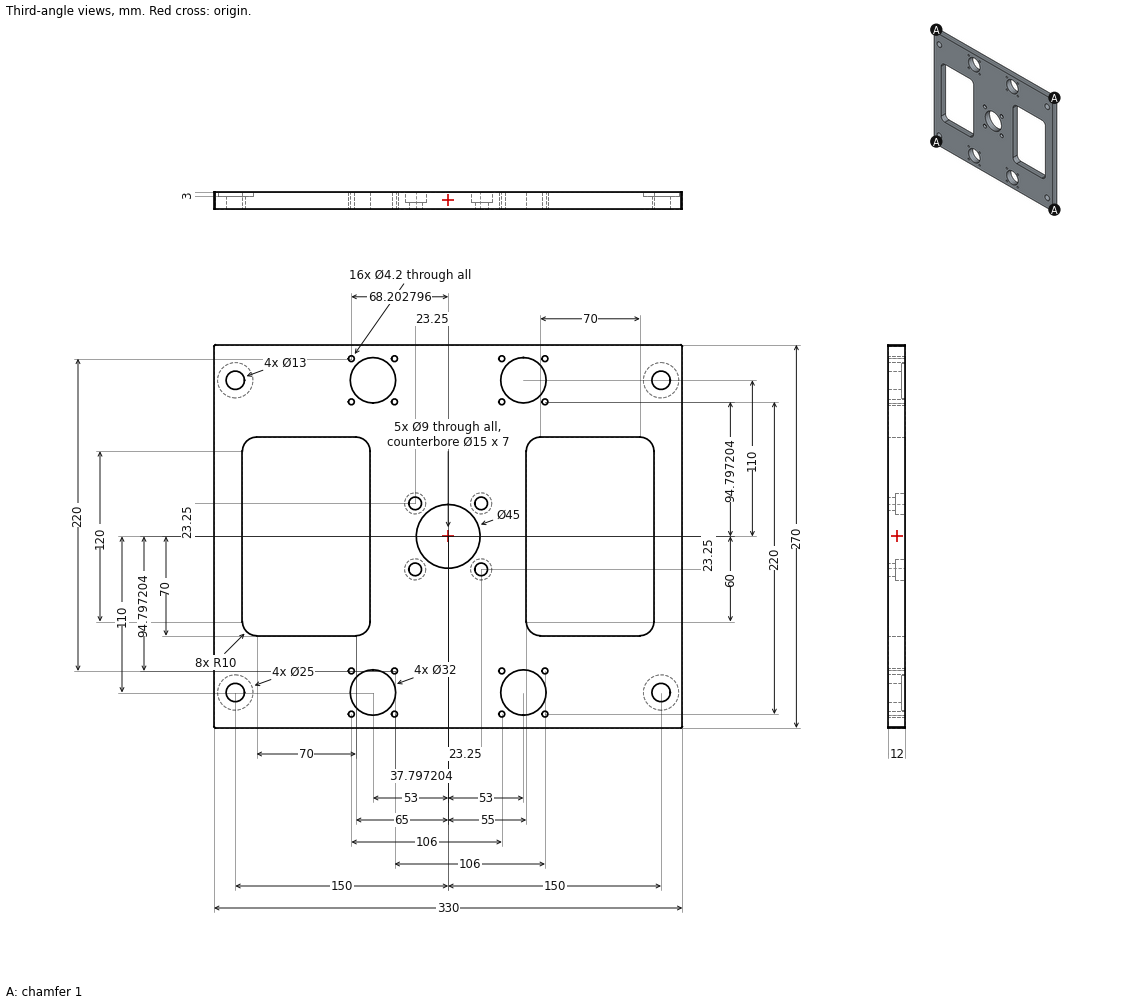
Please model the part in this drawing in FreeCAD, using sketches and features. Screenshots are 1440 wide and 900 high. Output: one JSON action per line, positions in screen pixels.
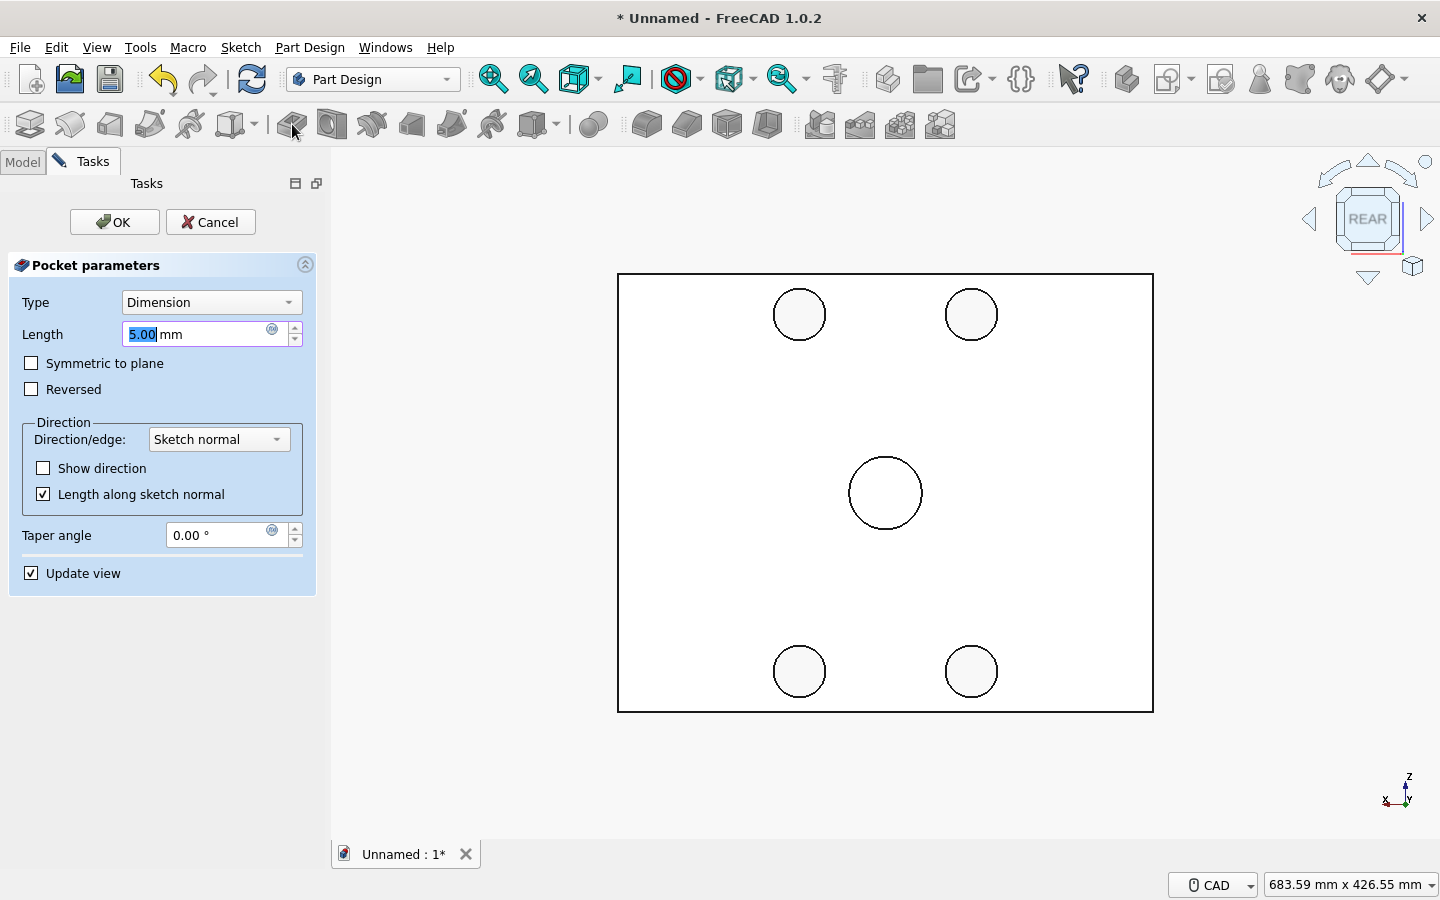
{"action": "left_click", "coordinate": [212, 302]}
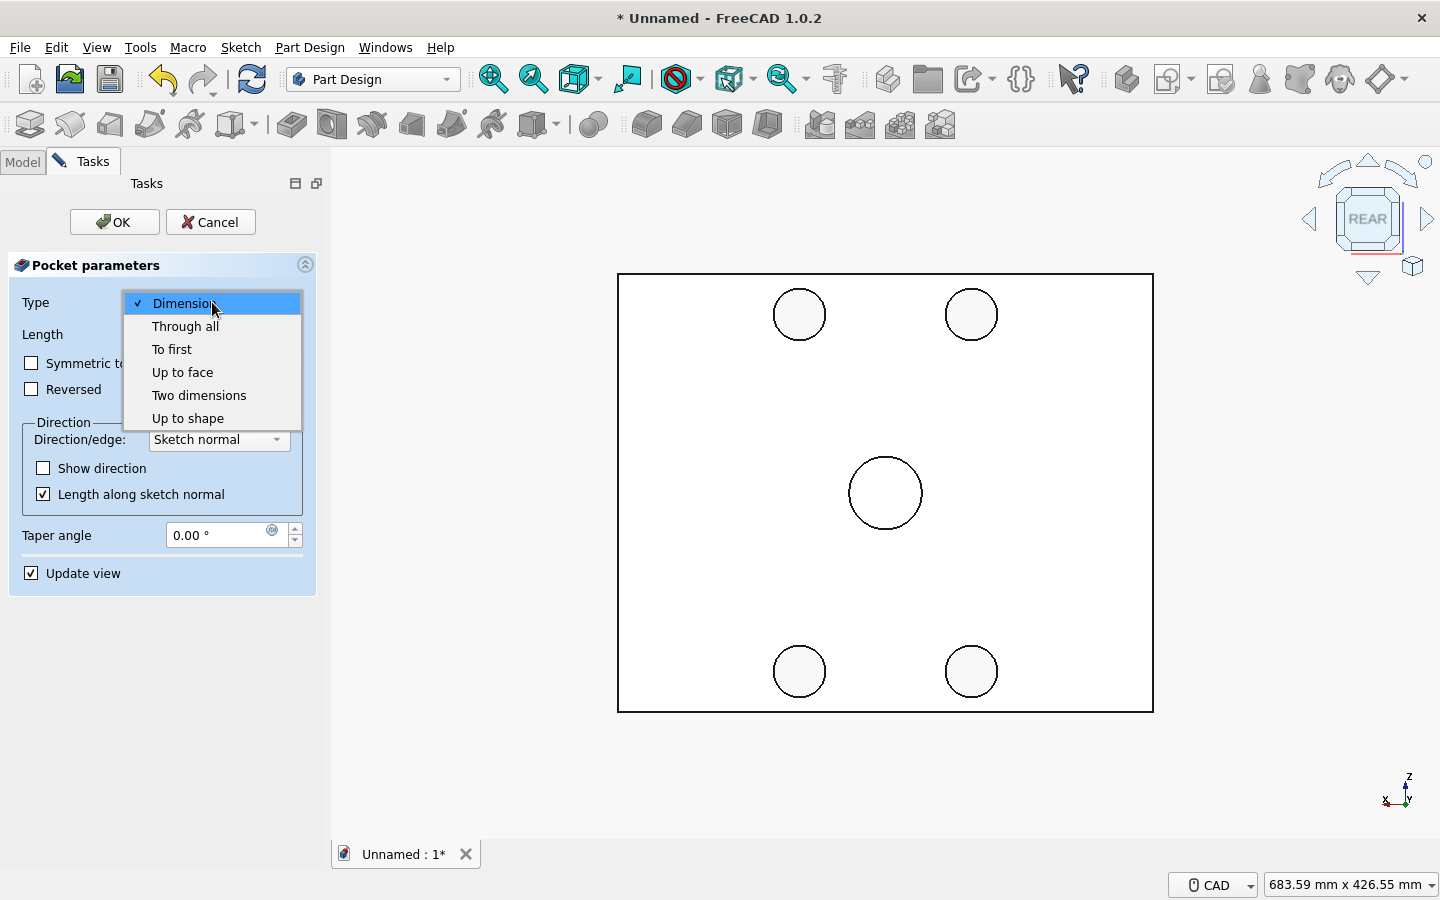
{"action": "left_click", "coordinate": [212, 326]}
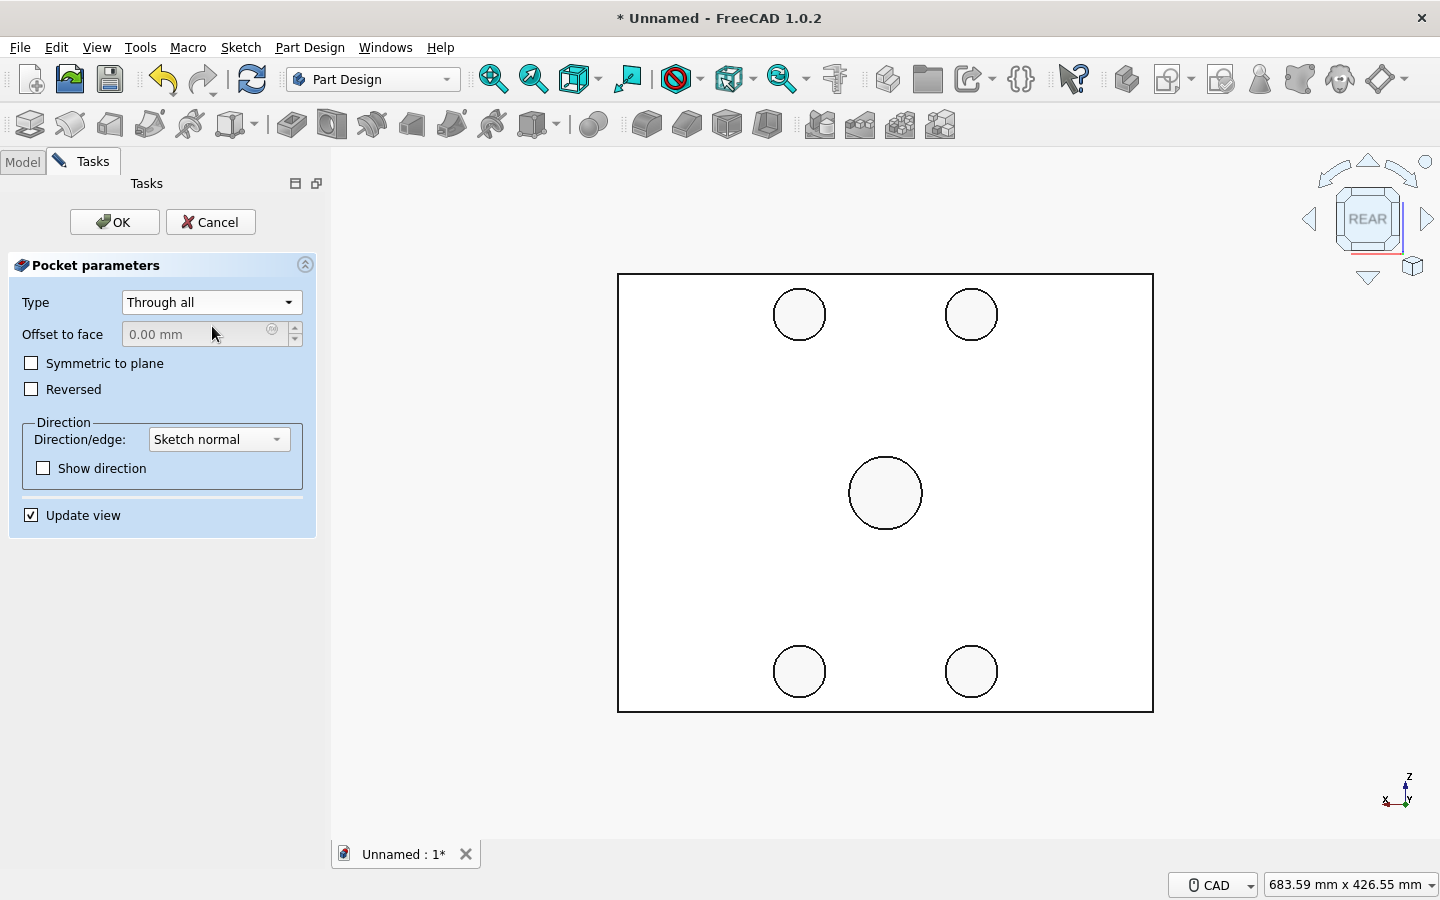
{"action": "left_click", "coordinate": [115, 222]}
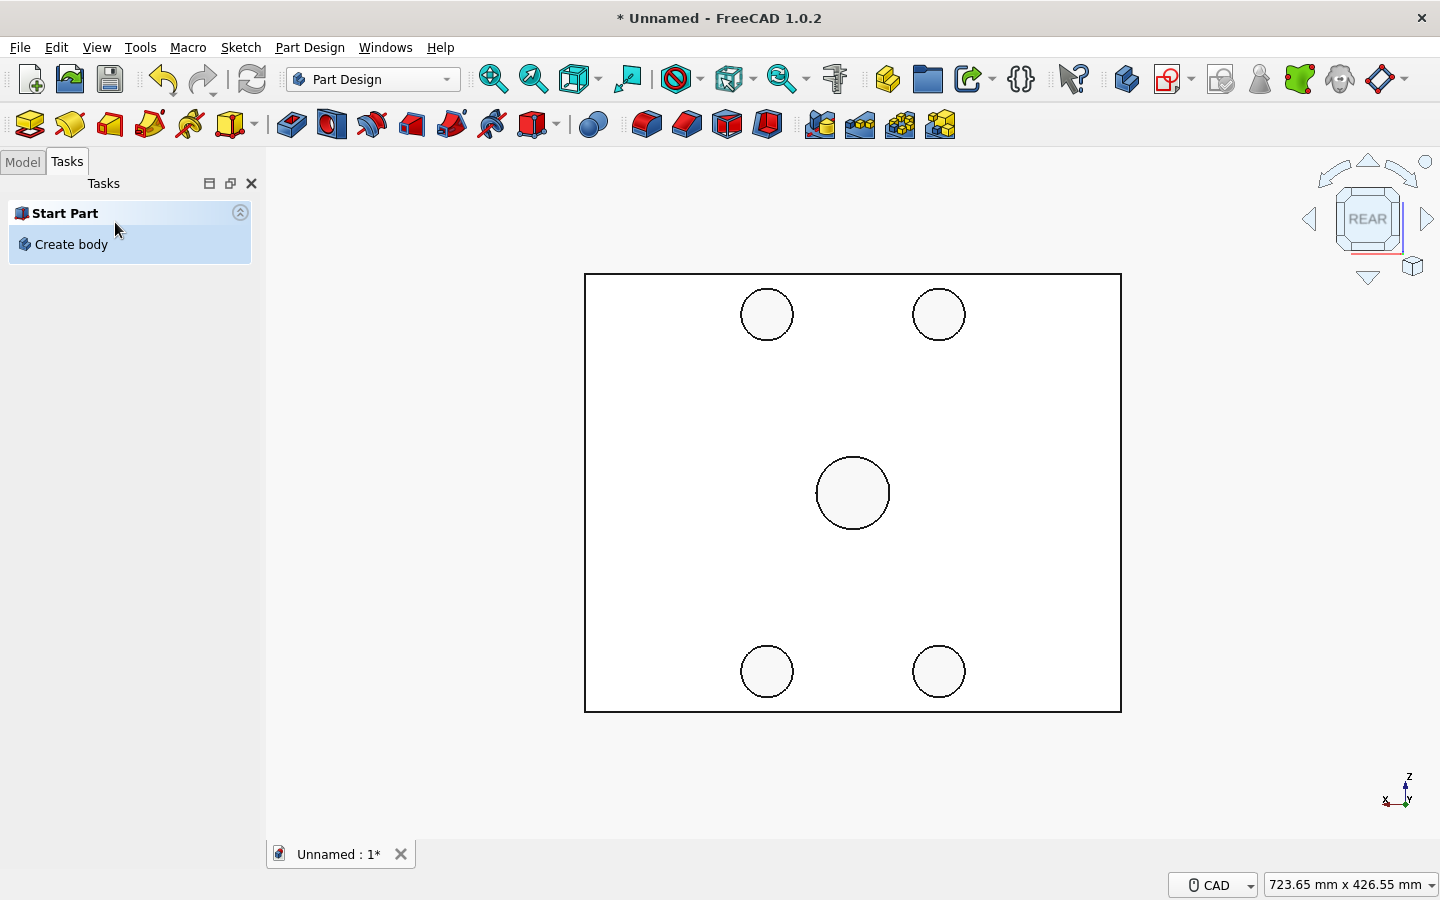
{"action": "left_click", "coordinate": [700, 492]}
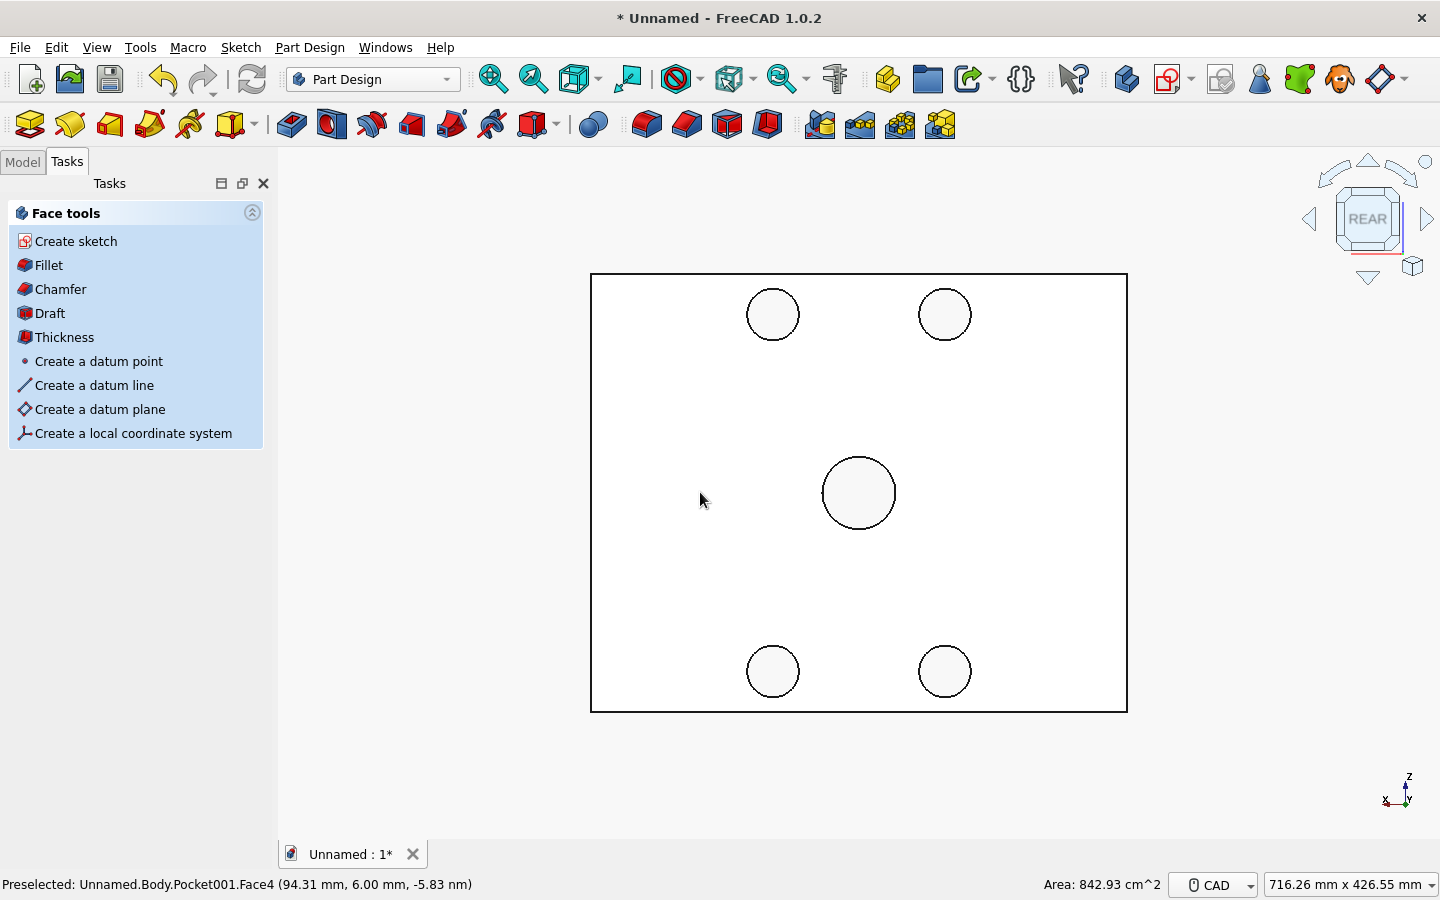
{"action": "left_click", "coordinate": [1168, 80]}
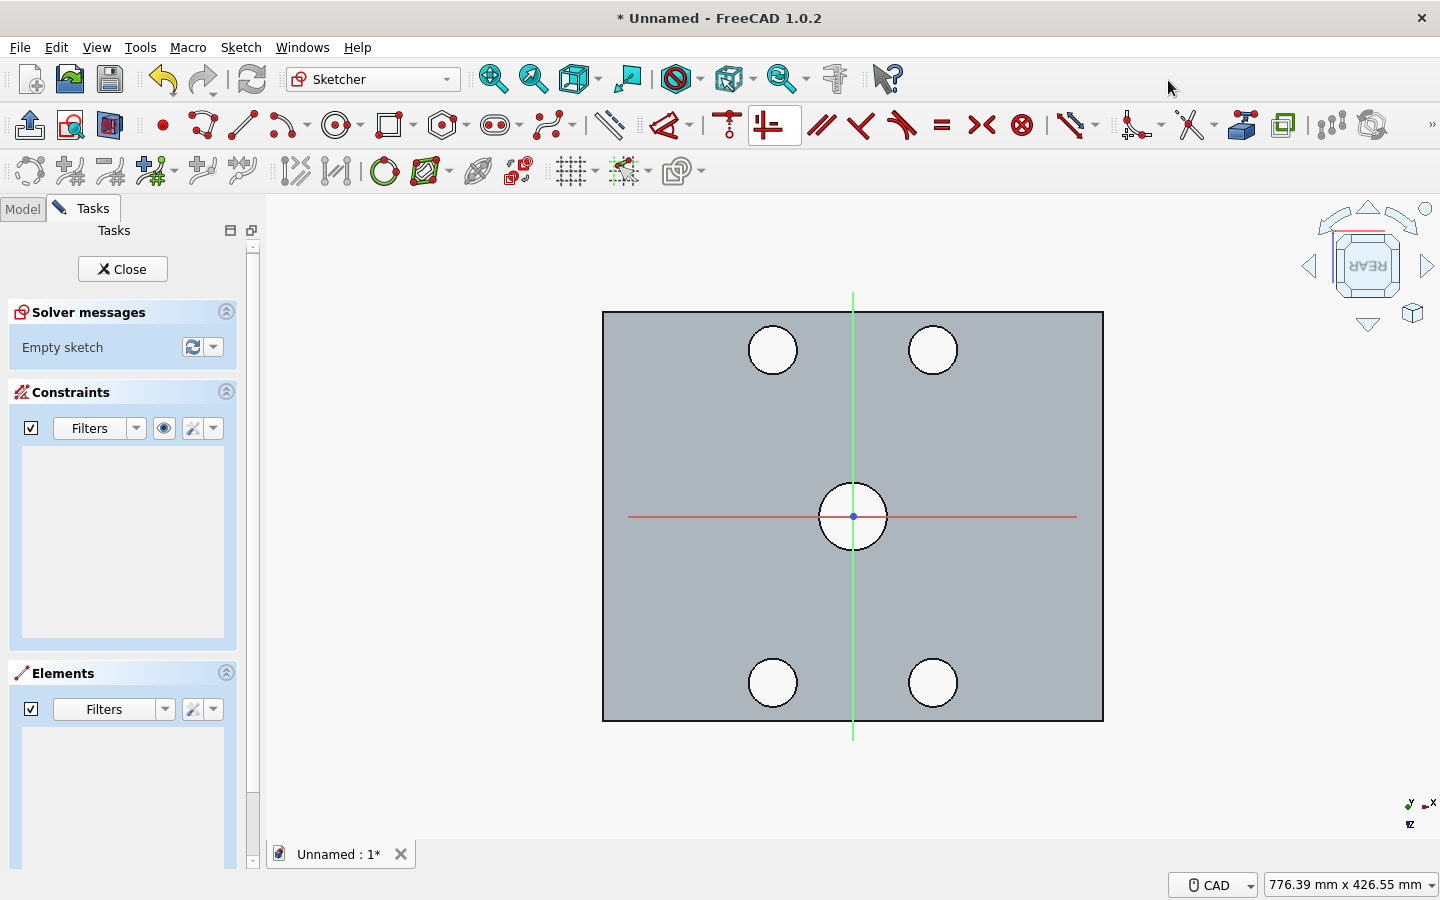
{"action": "key", "text": "g c"}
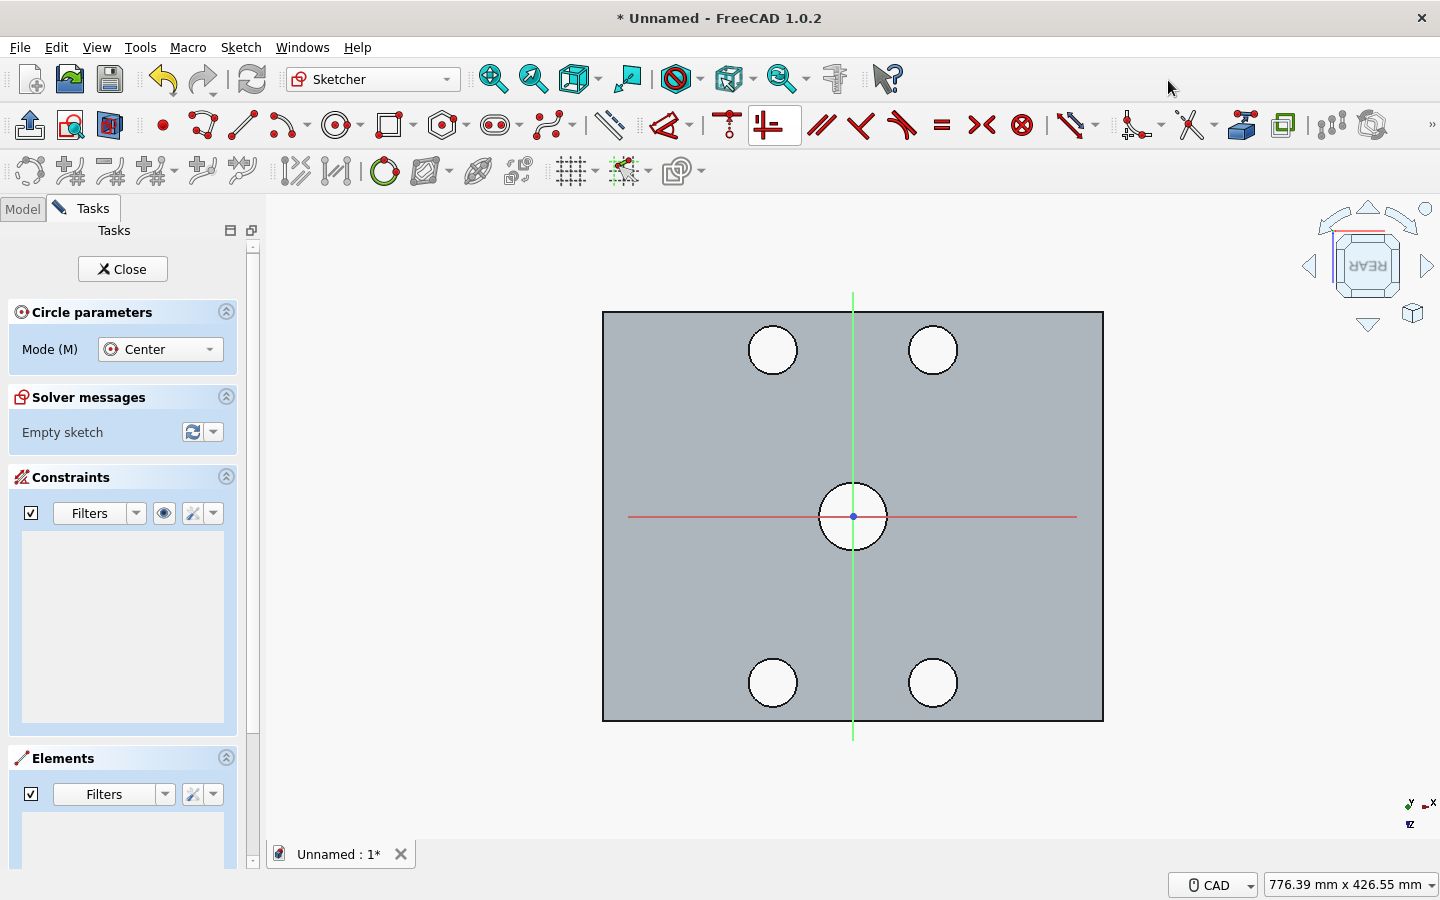
{"action": "left_click", "coordinate": [626, 350]}
{"action": "mouse_move", "coordinate": [640, 337]}